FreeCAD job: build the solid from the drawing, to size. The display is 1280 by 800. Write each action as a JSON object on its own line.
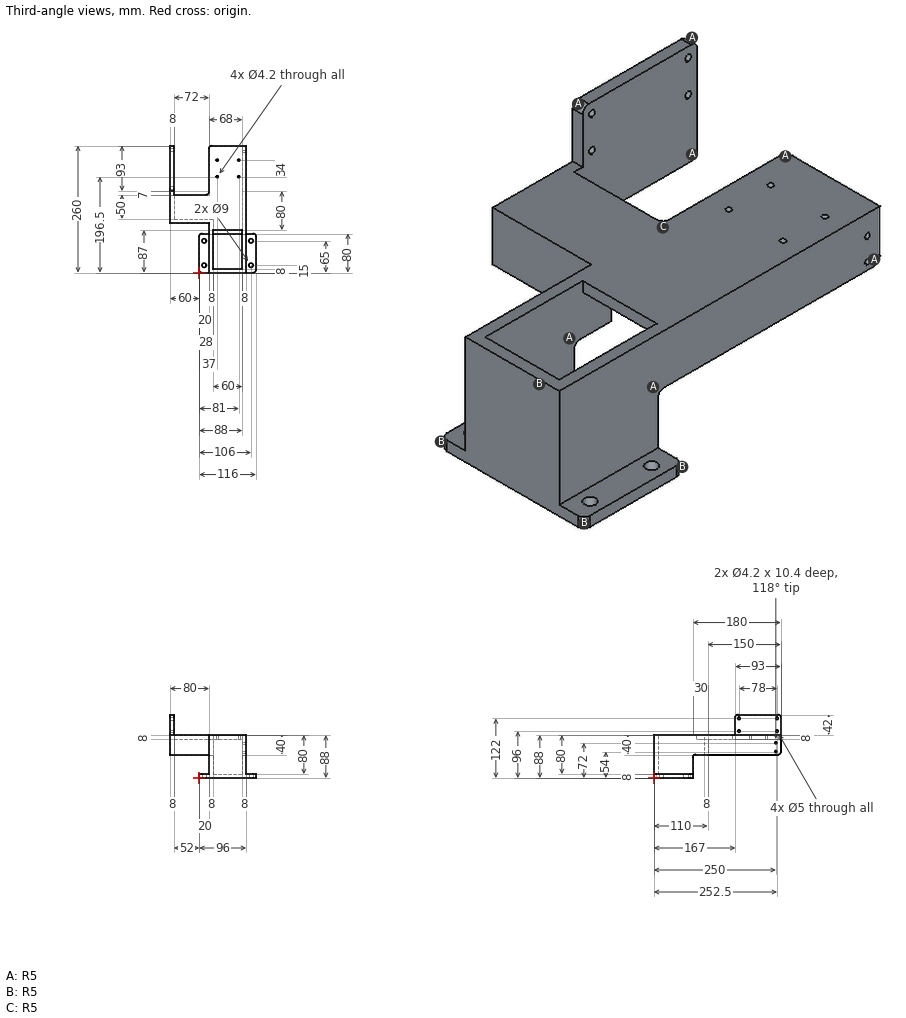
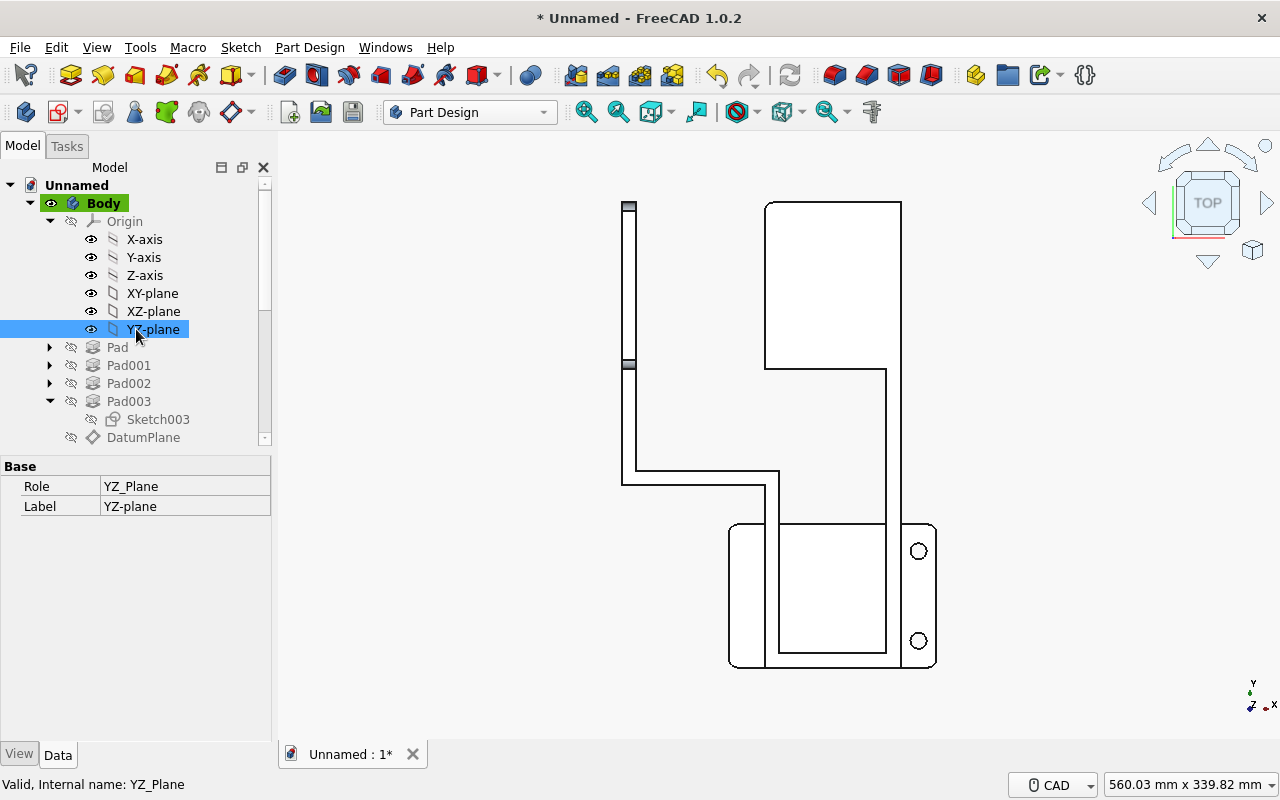
{"action": "left_click", "coordinate": [232, 112]}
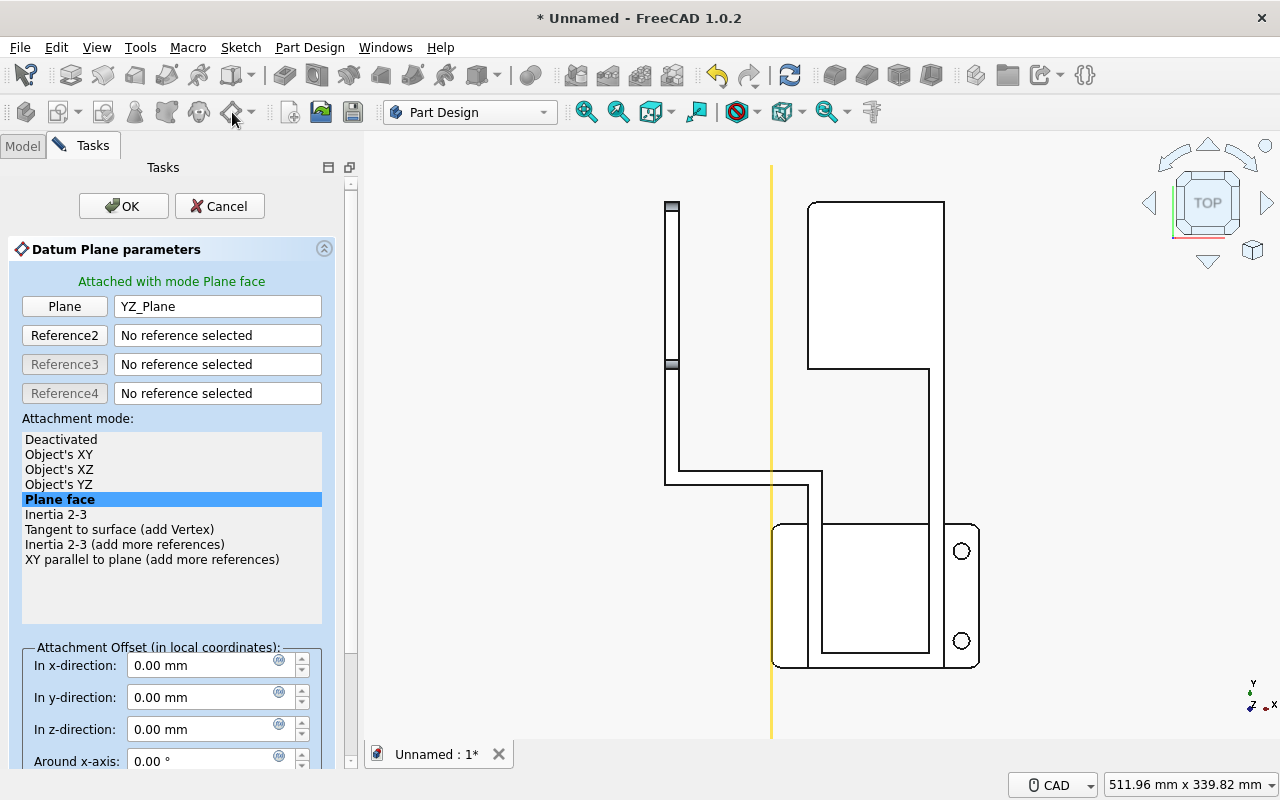
{"action": "triple_click", "coordinate": [210, 729]}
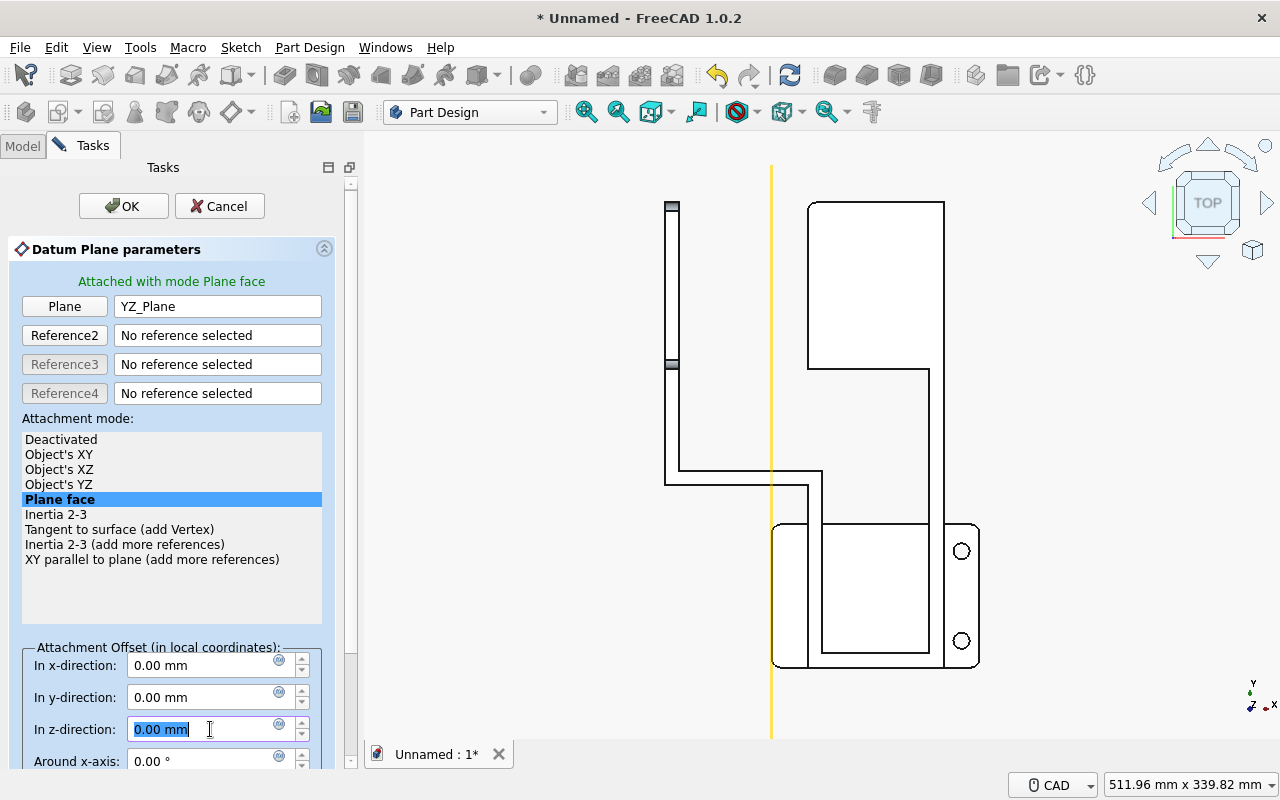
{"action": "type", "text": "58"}
{"action": "key", "text": "Tab"}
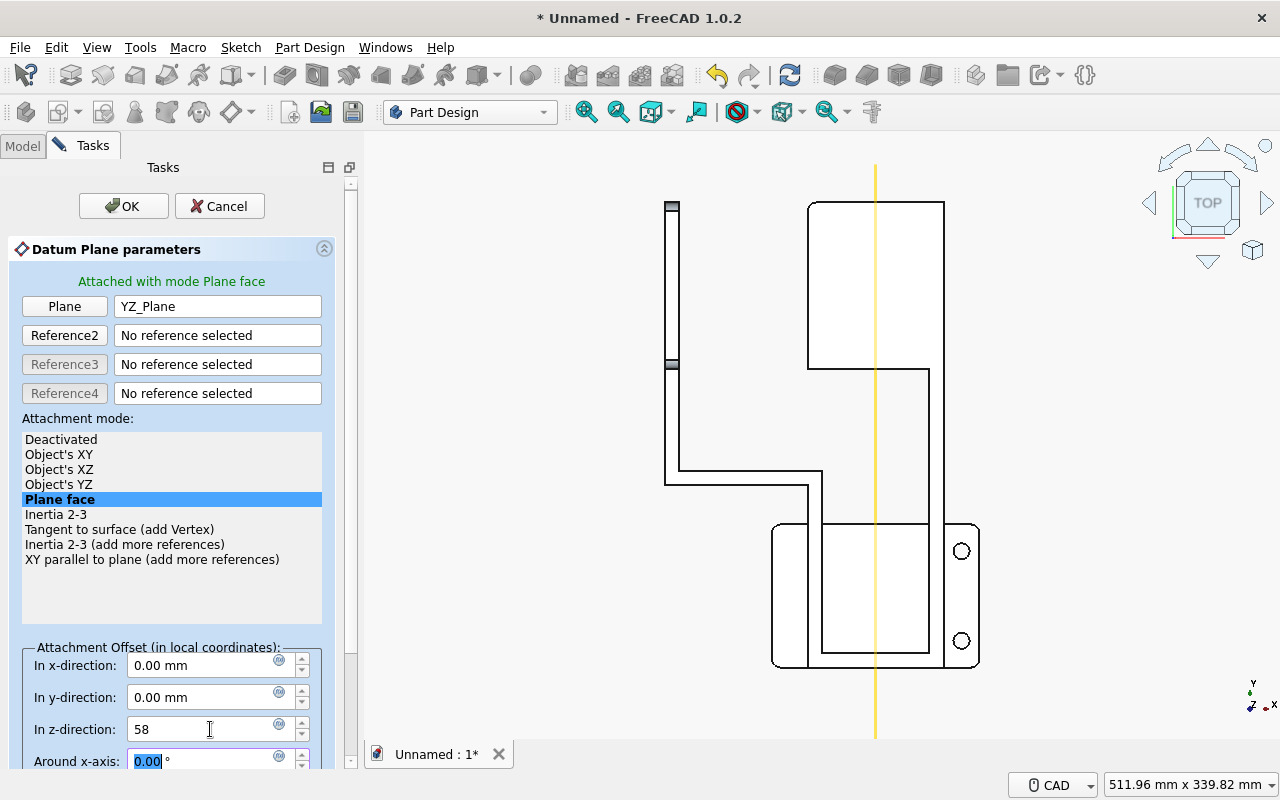
{"action": "left_click", "coordinate": [124, 206]}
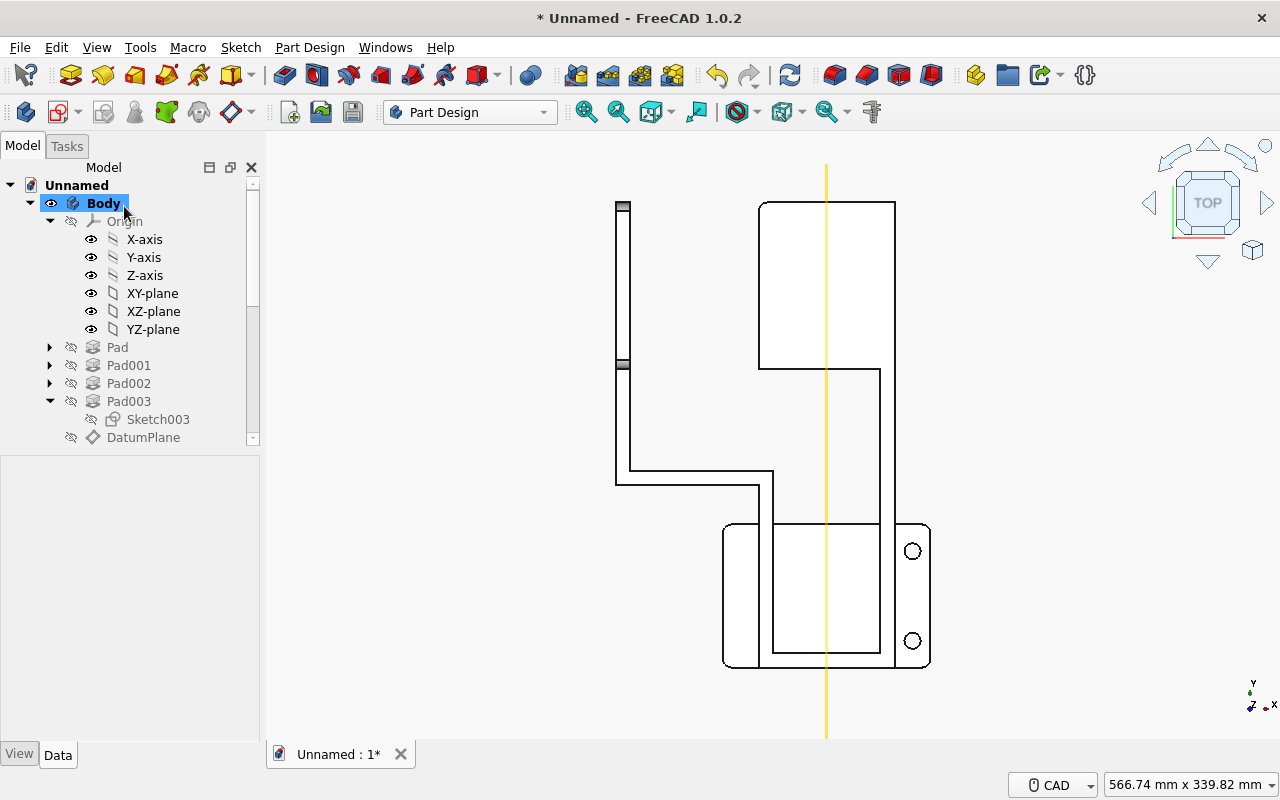
{"action": "scroll", "coordinate": [100, 307], "scroll_direction": "down", "scroll_amount": 3}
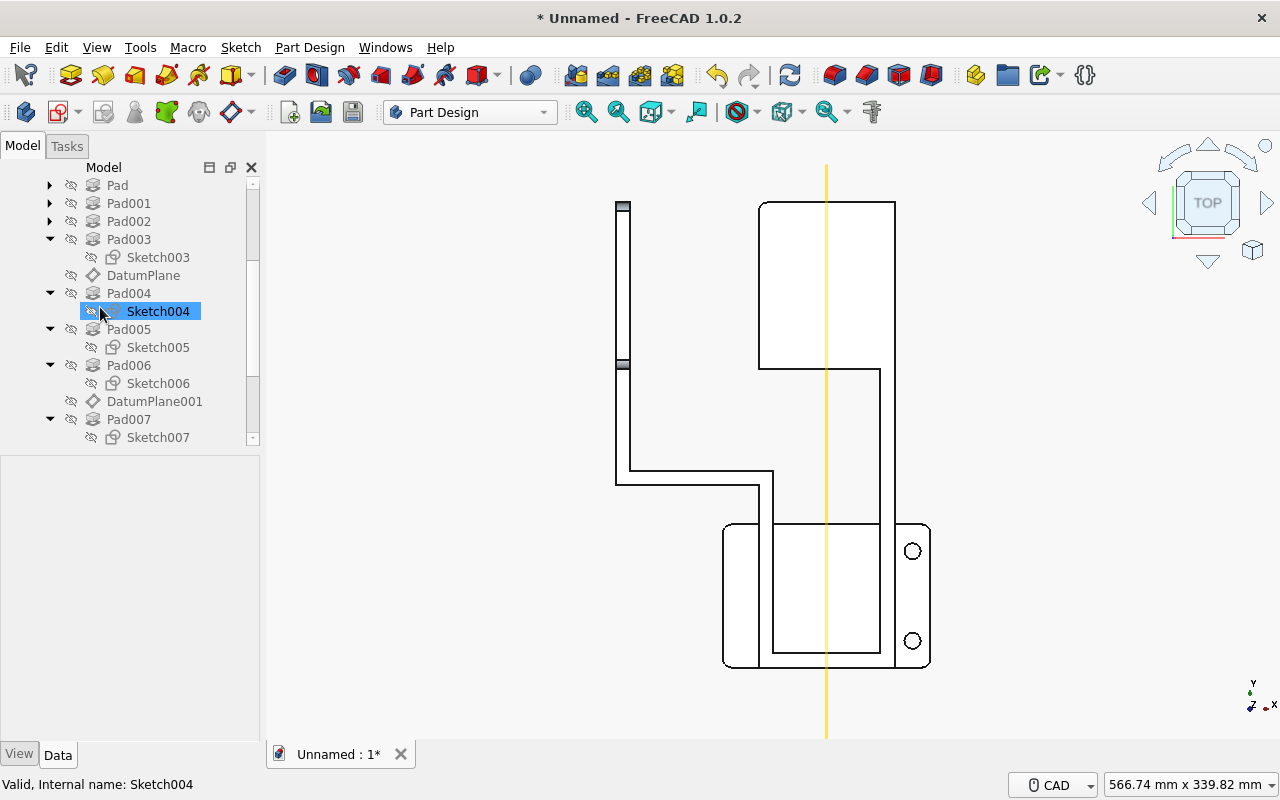
{"action": "scroll", "coordinate": [140, 307], "scroll_direction": "up", "scroll_amount": 15}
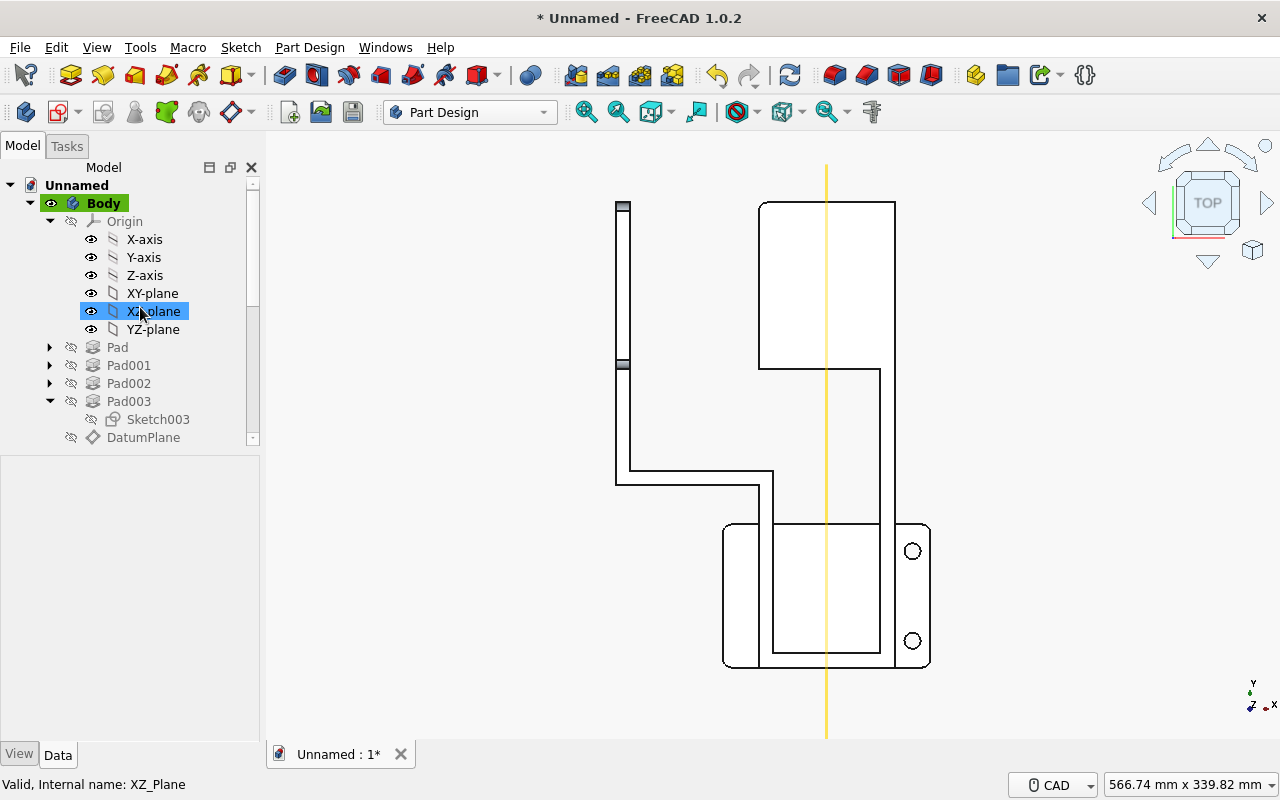
{"action": "scroll", "coordinate": [100, 307], "scroll_direction": "down", "scroll_amount": 6}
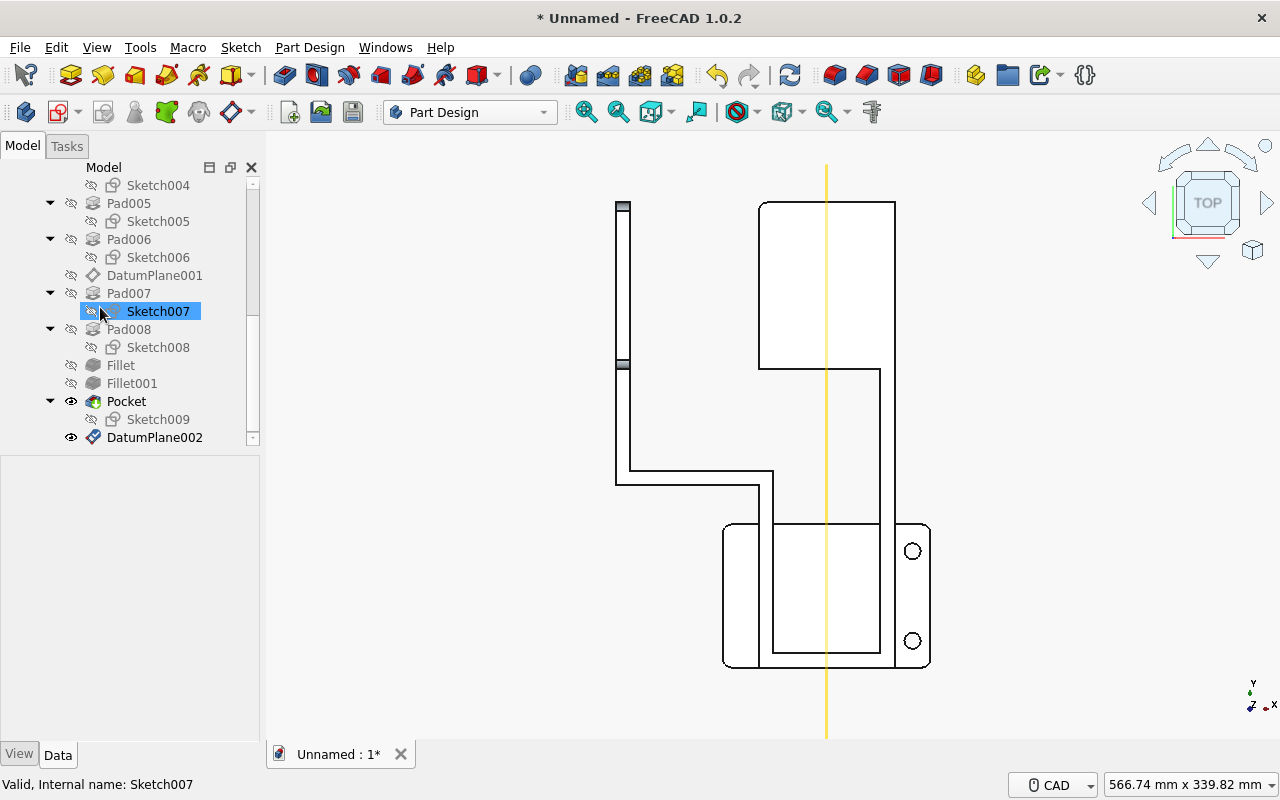
{"action": "left_click", "coordinate": [116, 401]}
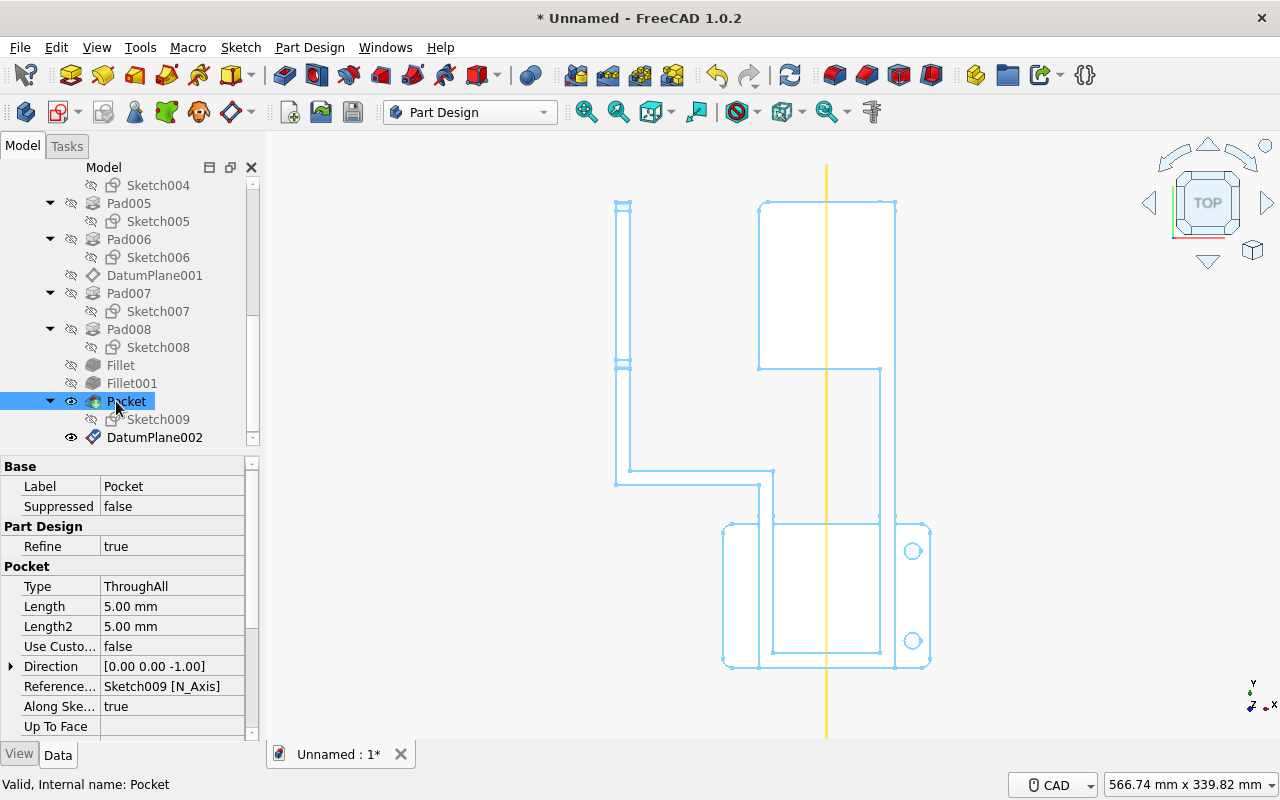
{"action": "left_click", "coordinate": [576, 76]}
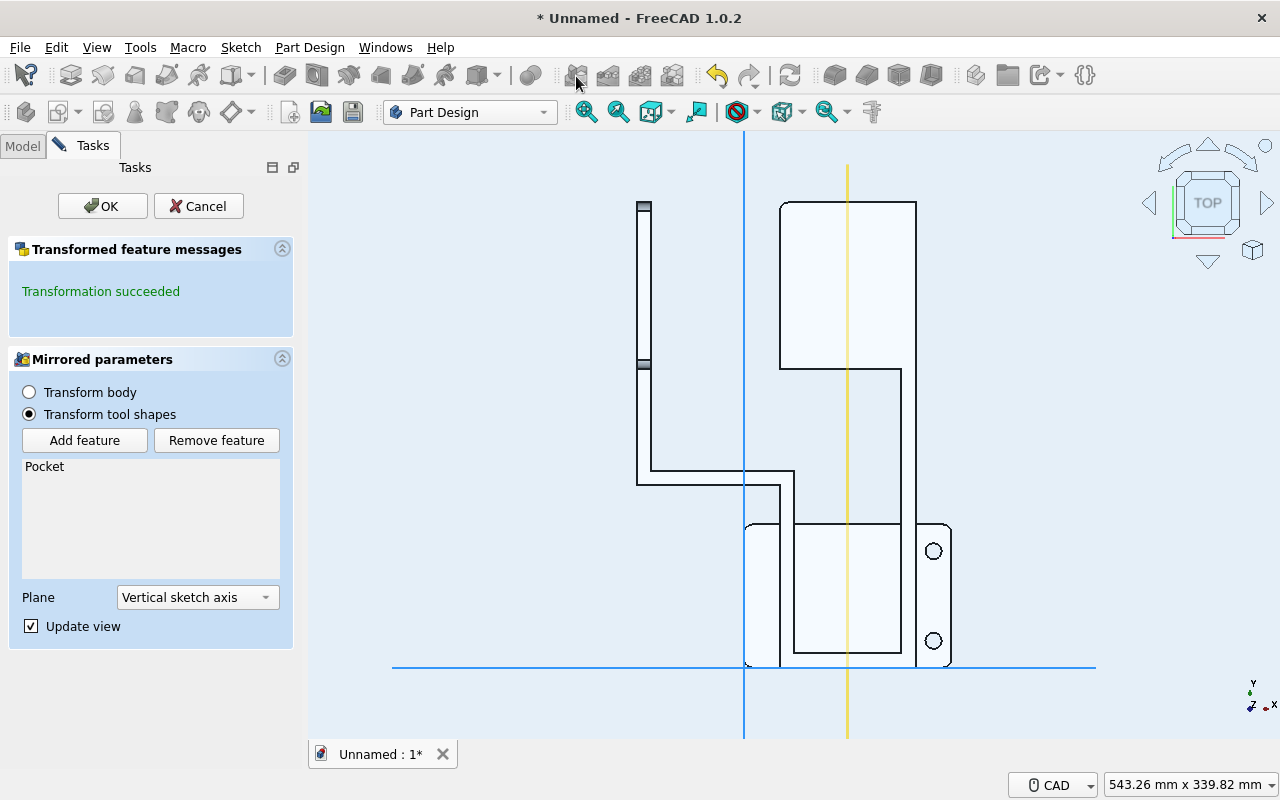
{"action": "left_click", "coordinate": [198, 598]}